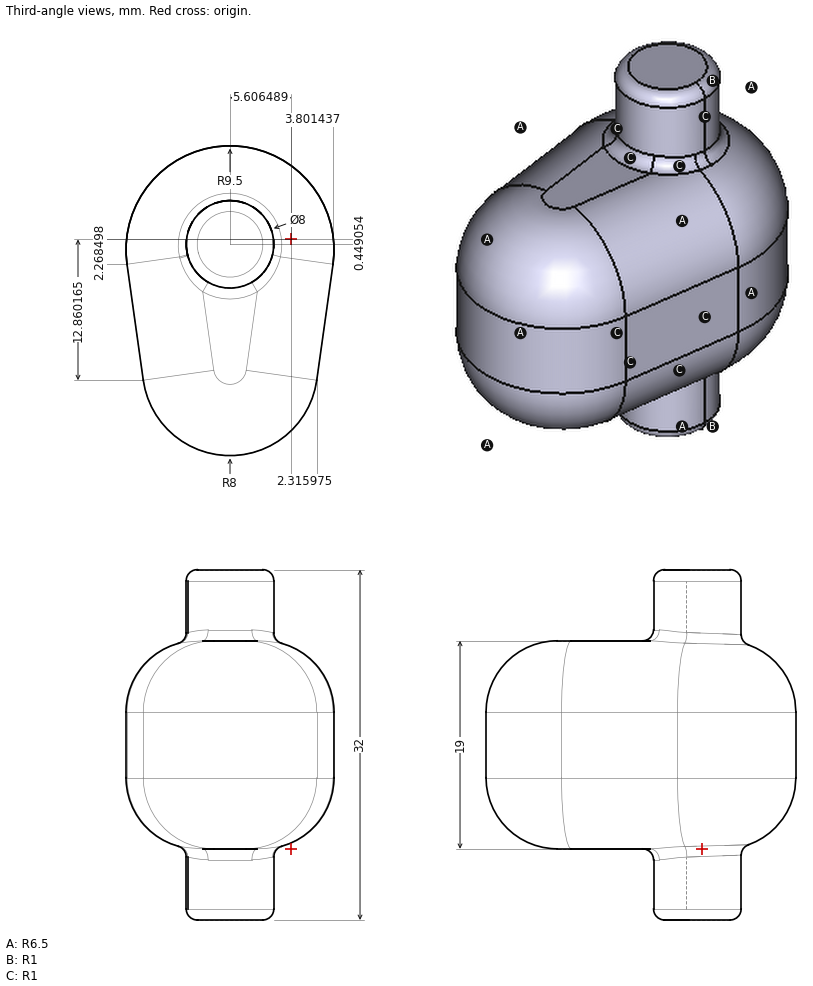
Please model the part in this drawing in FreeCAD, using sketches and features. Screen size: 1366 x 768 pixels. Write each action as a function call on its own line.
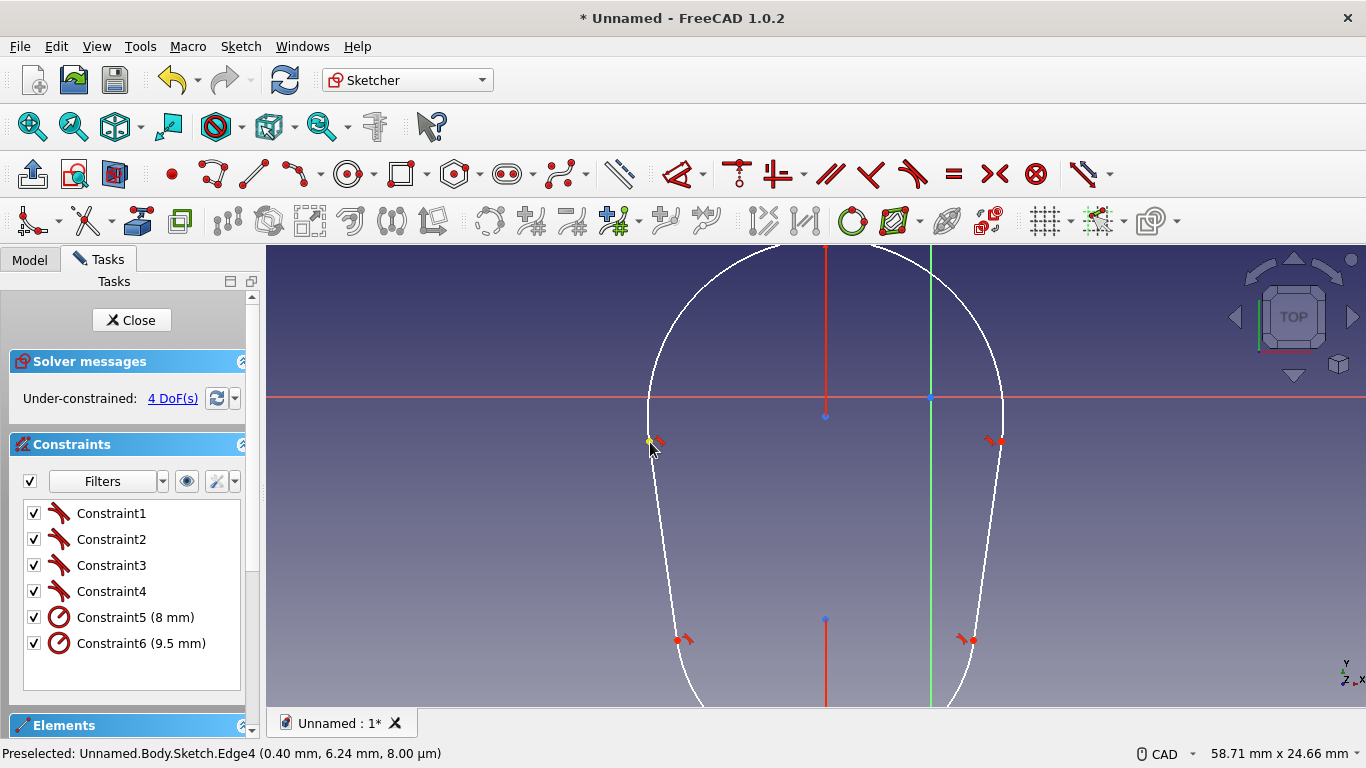
click(649, 442)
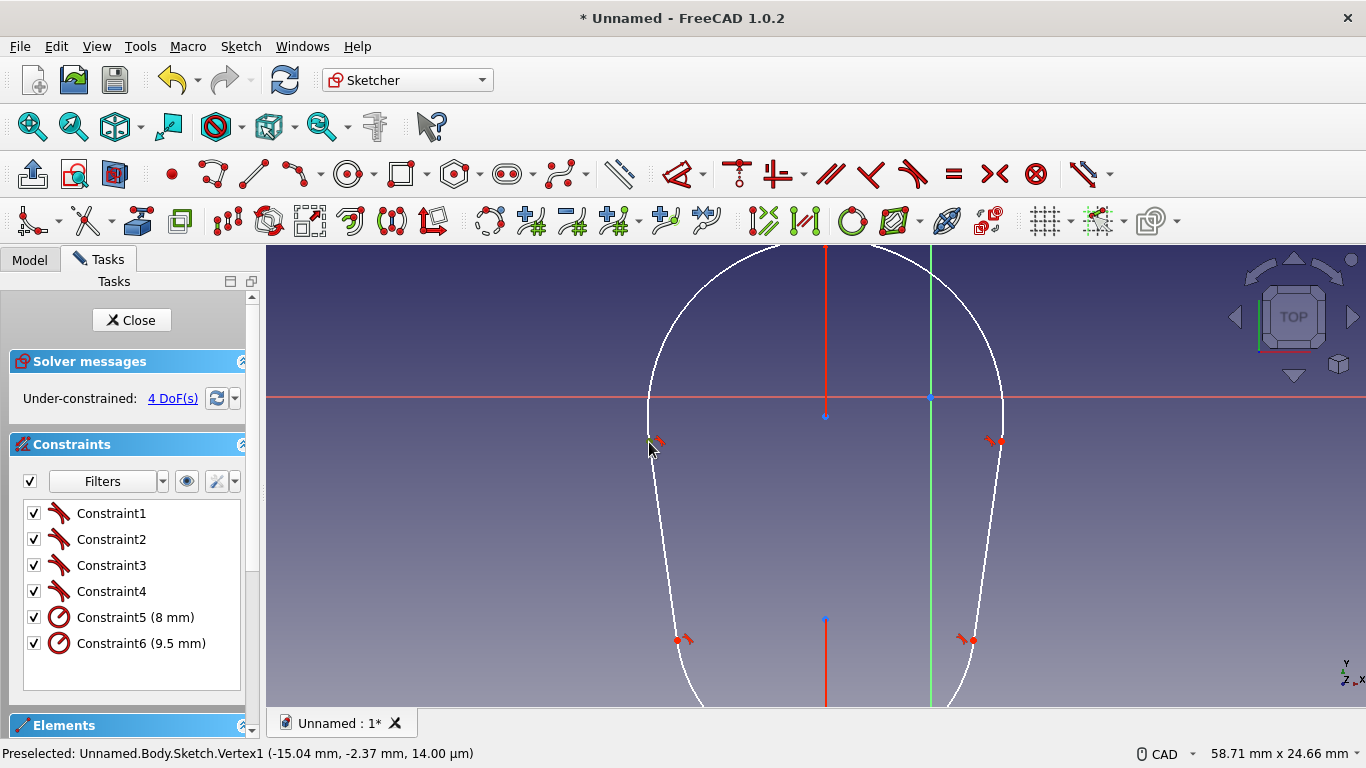
key(i)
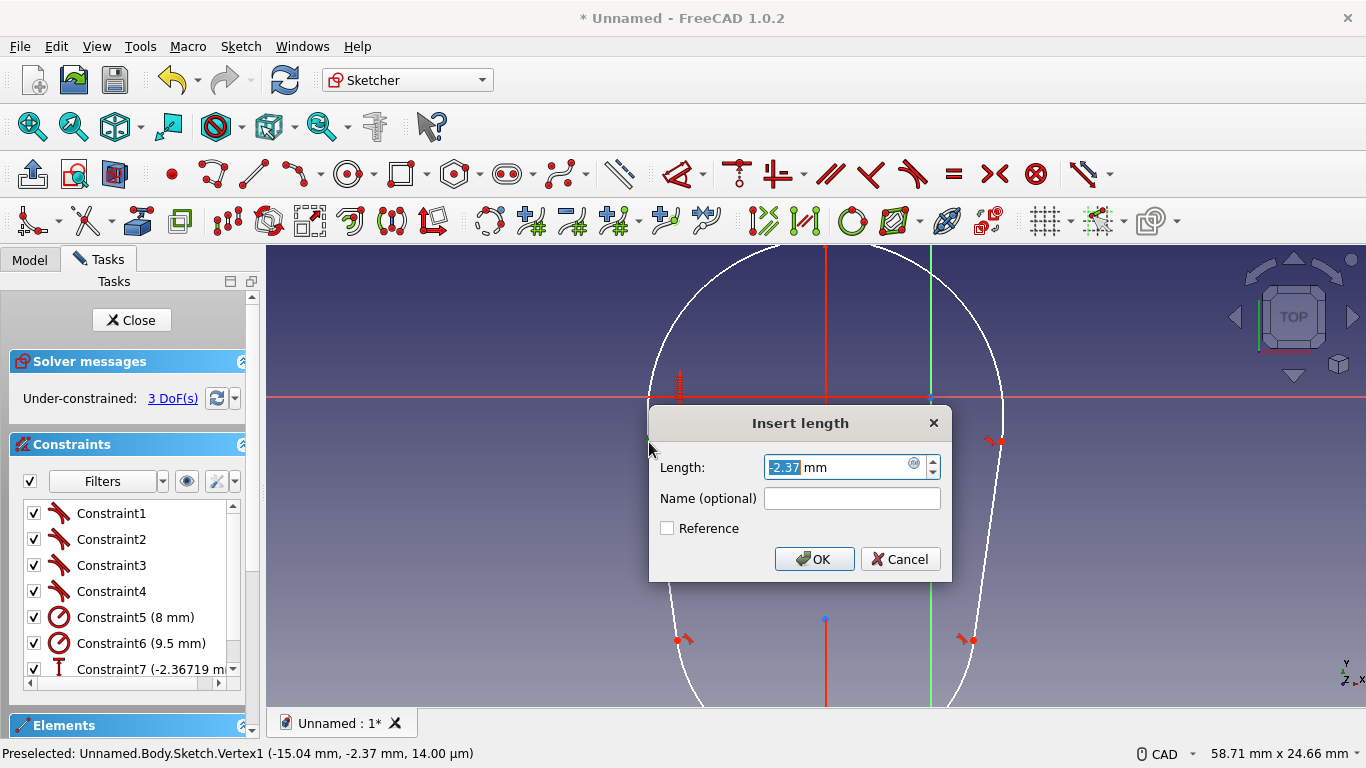
text(-2.268498)
key(Return)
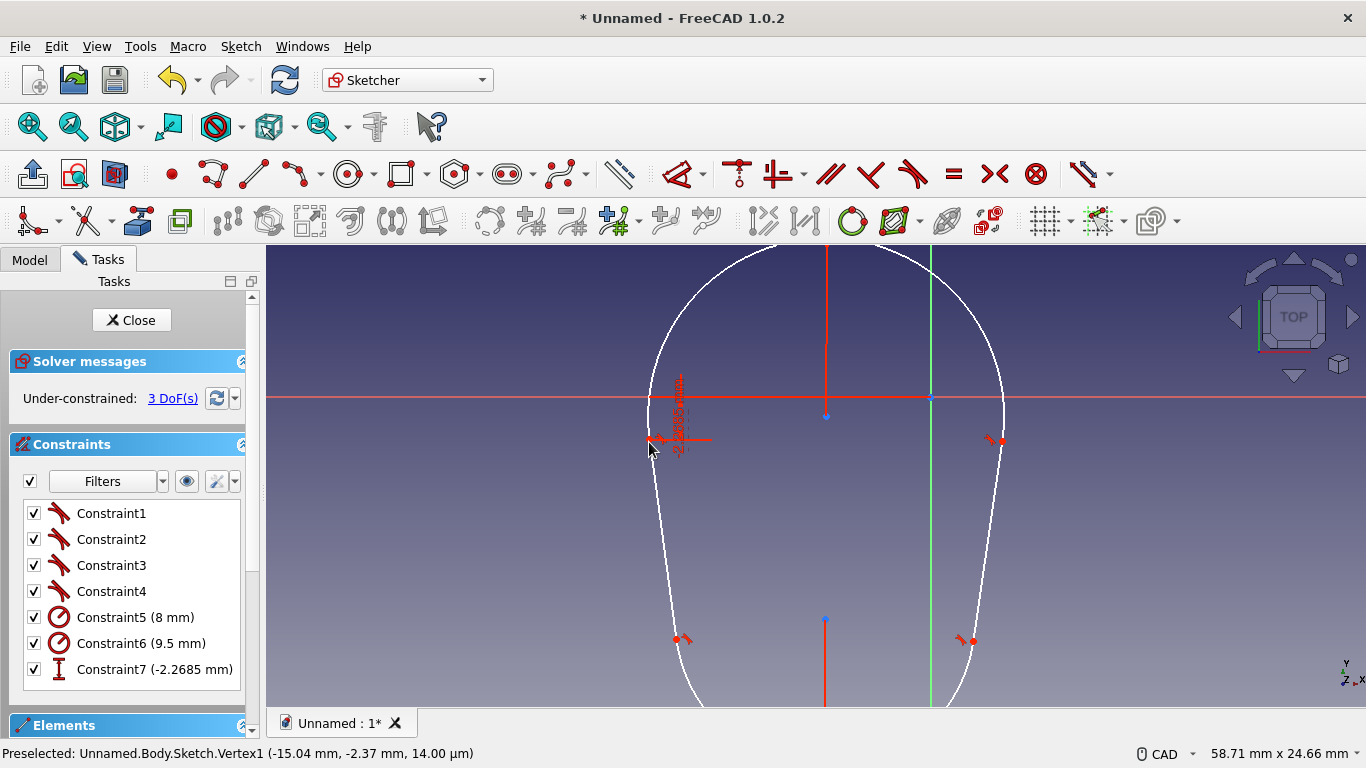
click(973, 641)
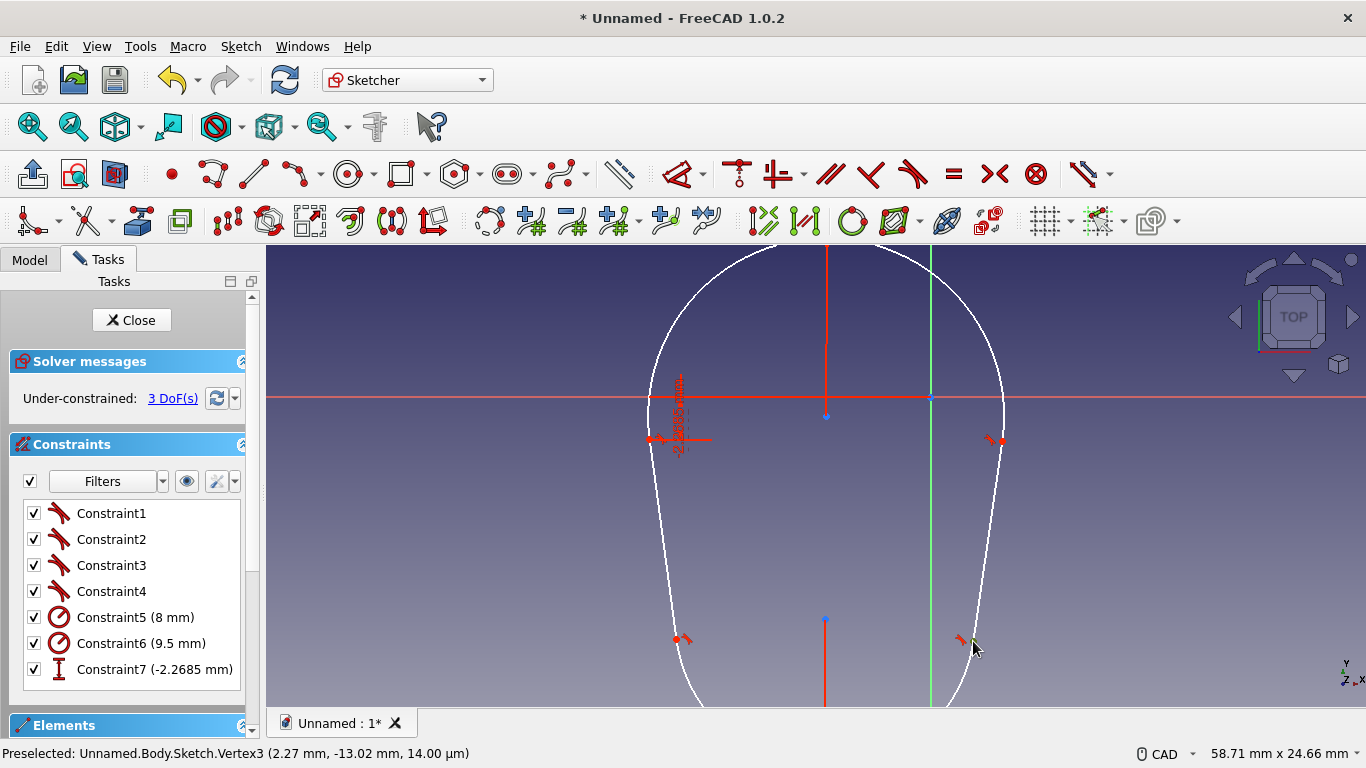
click(702, 174)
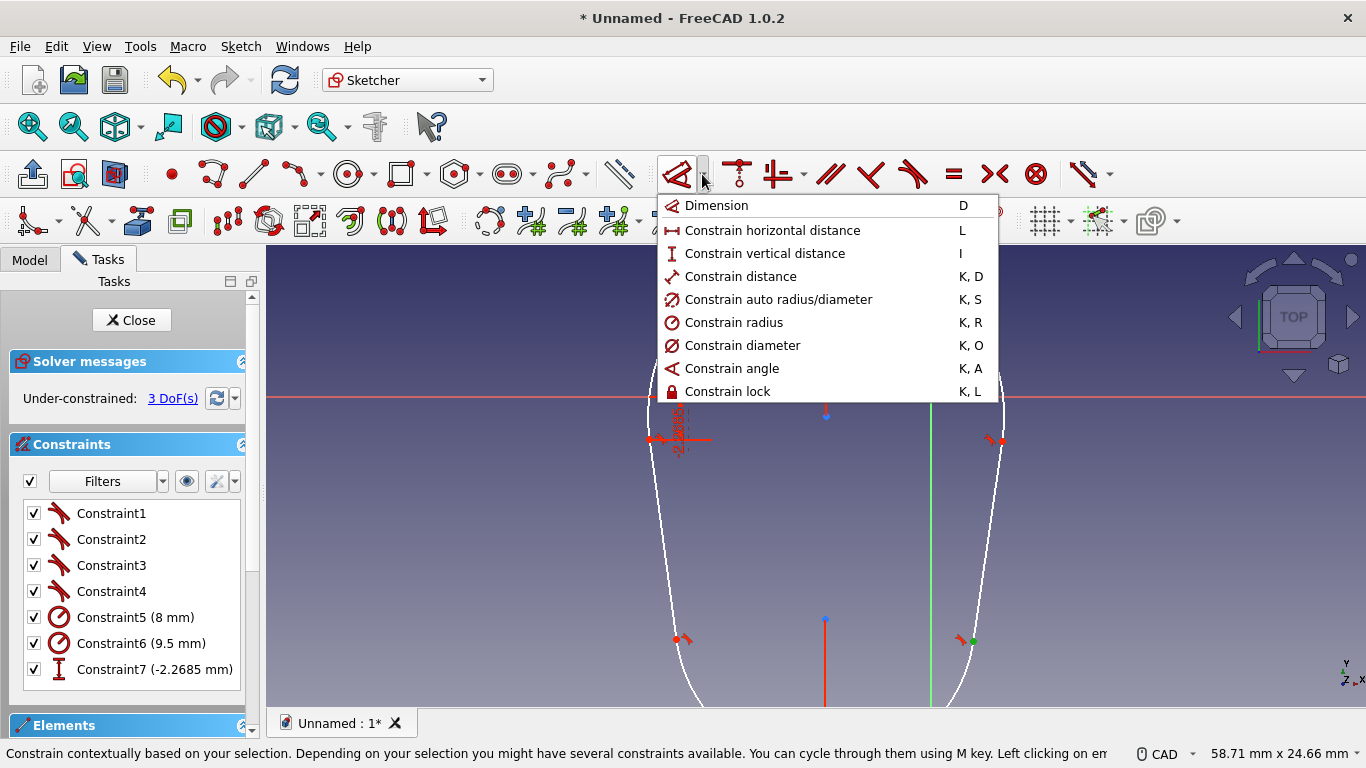
click(828, 230)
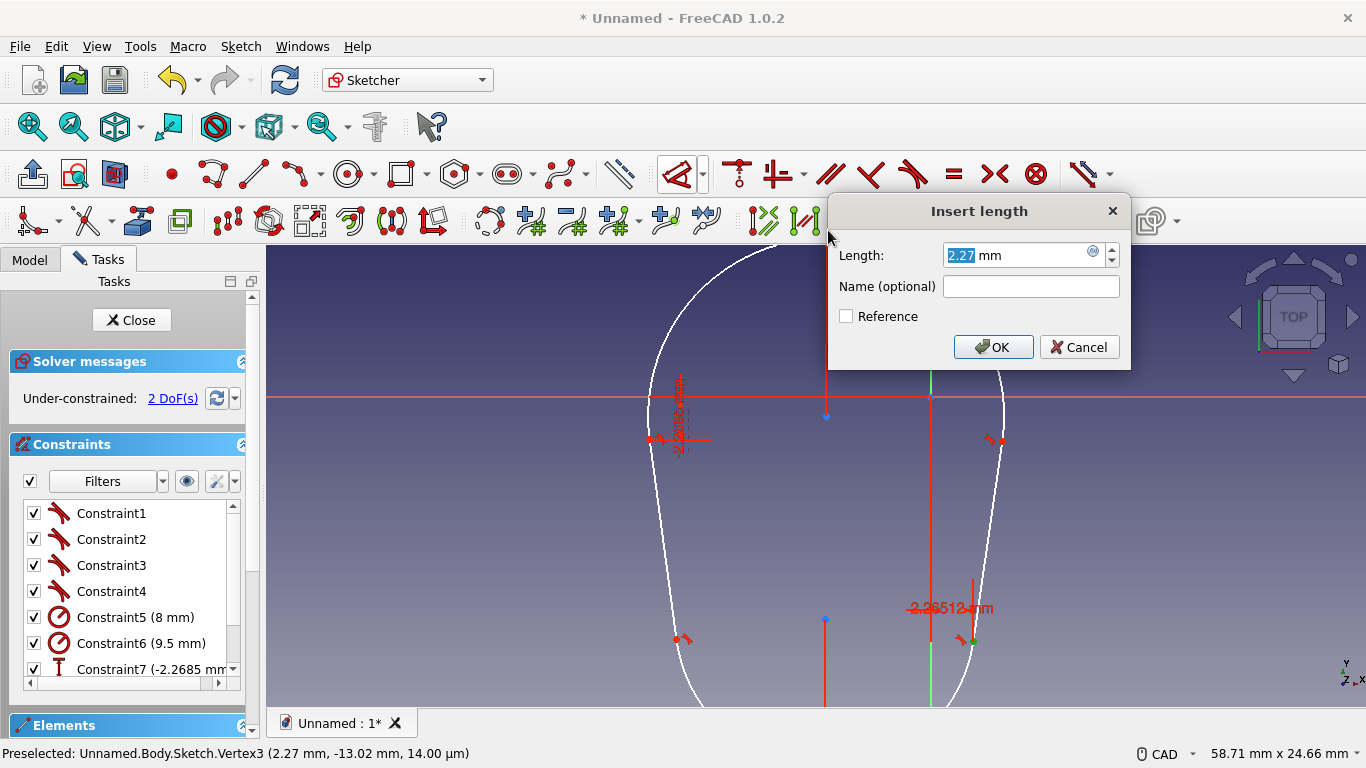
text(2.315975)
key(Return)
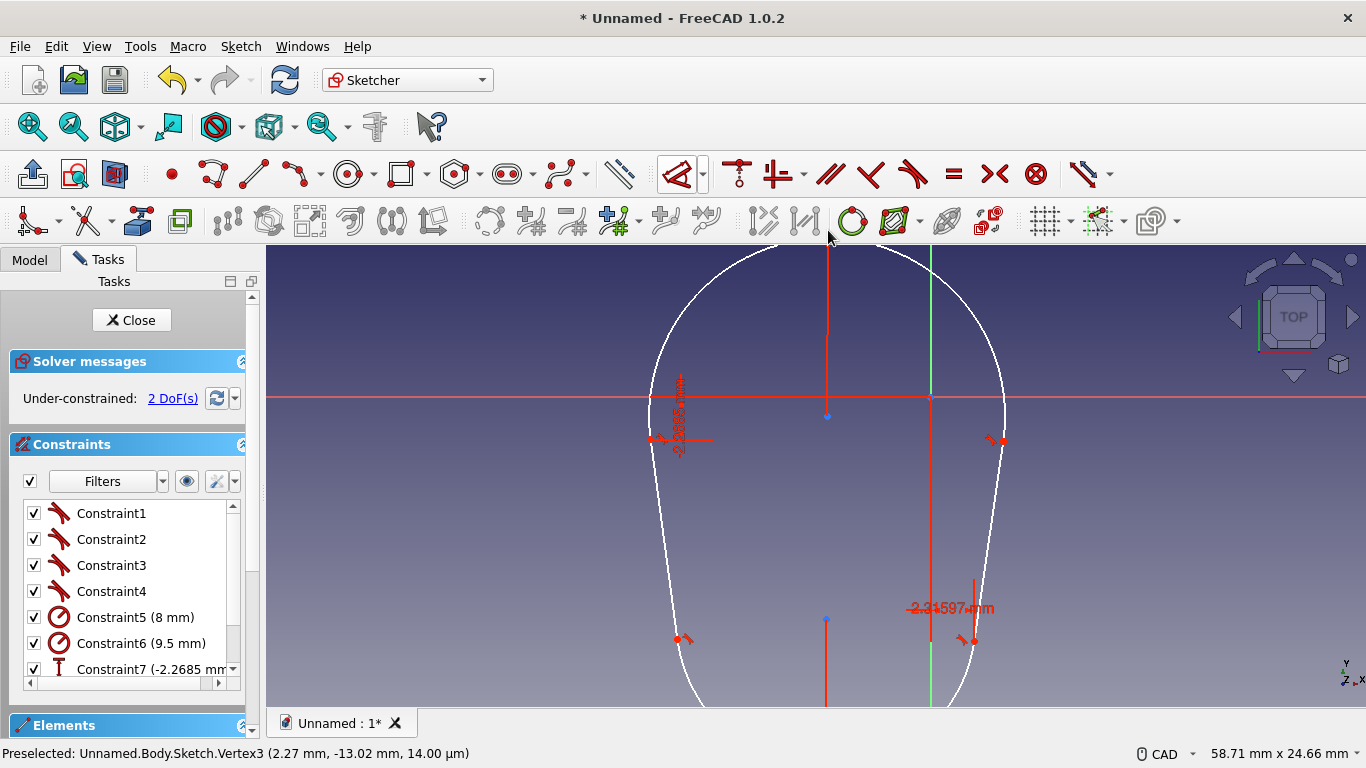
click(1003, 442)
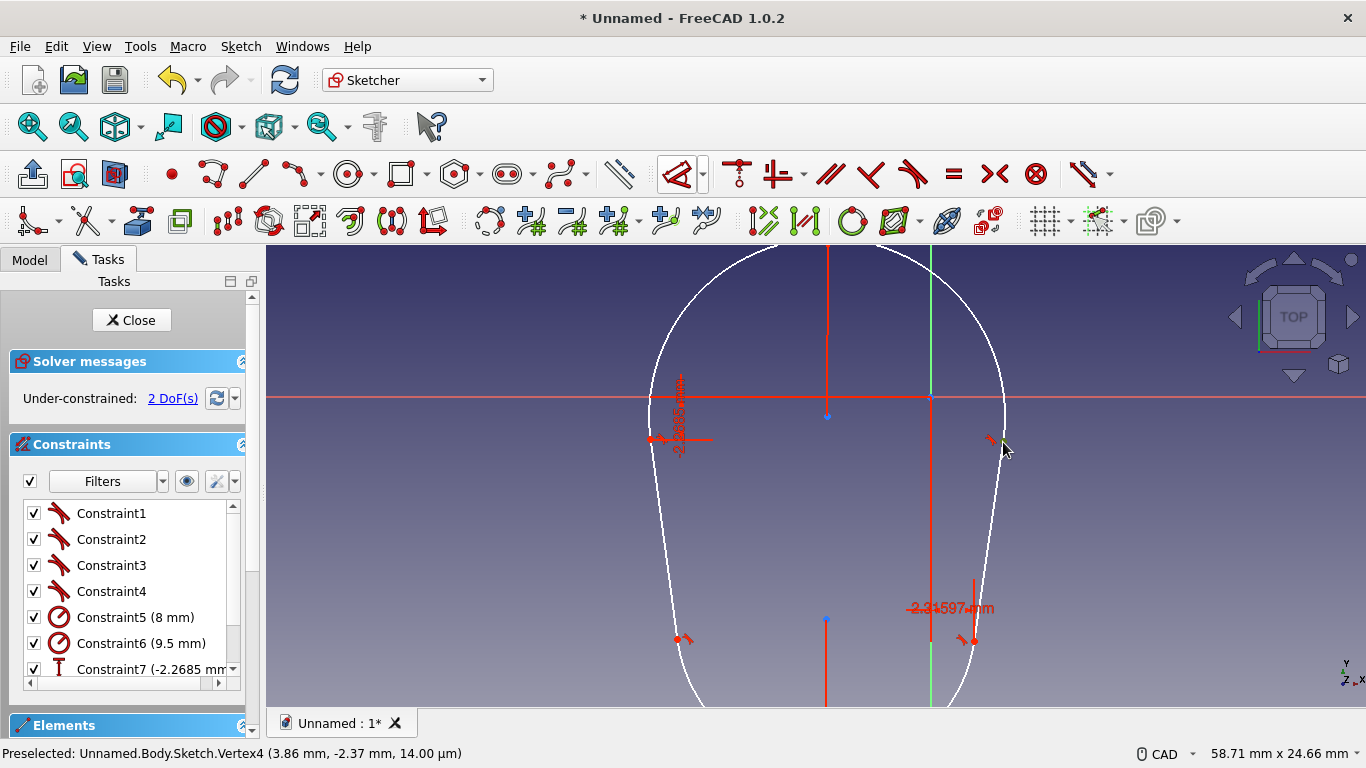
key(l)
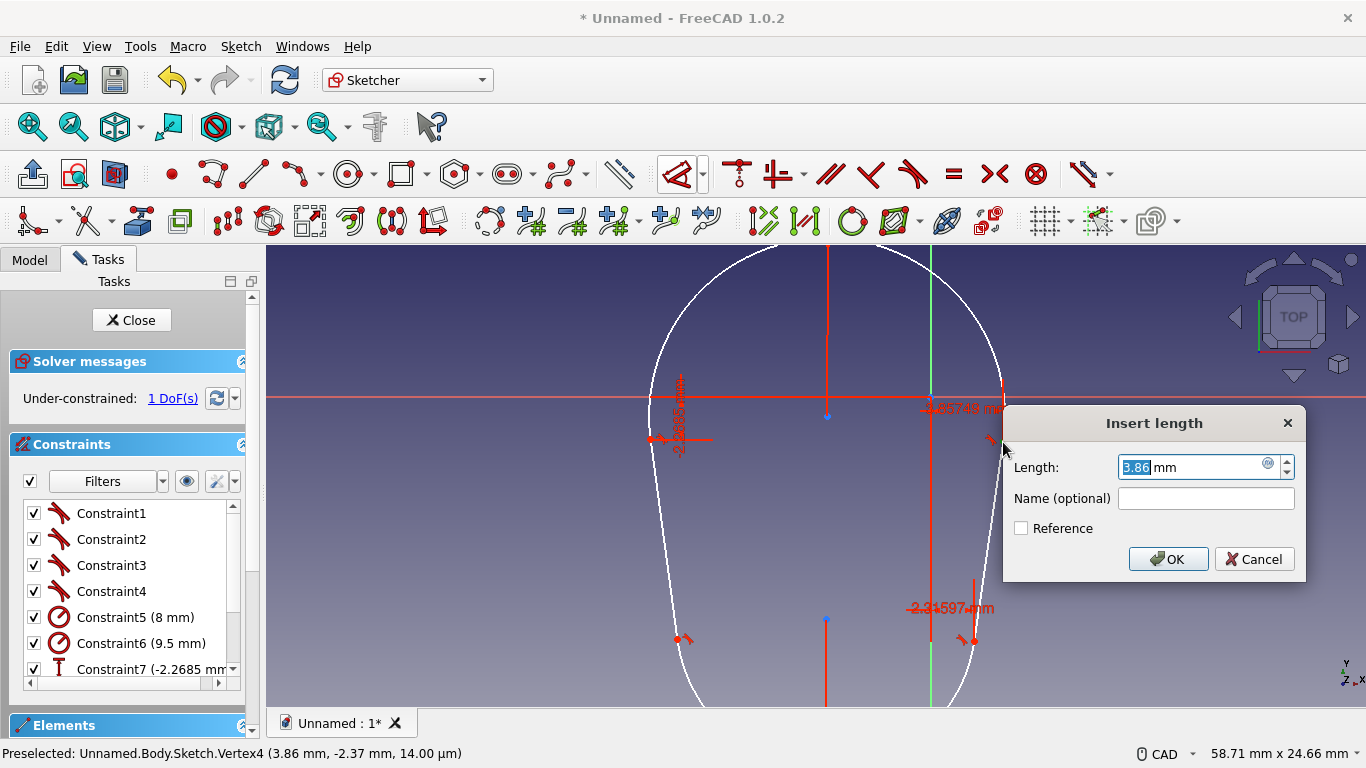
text(3.801437)
key(Return)